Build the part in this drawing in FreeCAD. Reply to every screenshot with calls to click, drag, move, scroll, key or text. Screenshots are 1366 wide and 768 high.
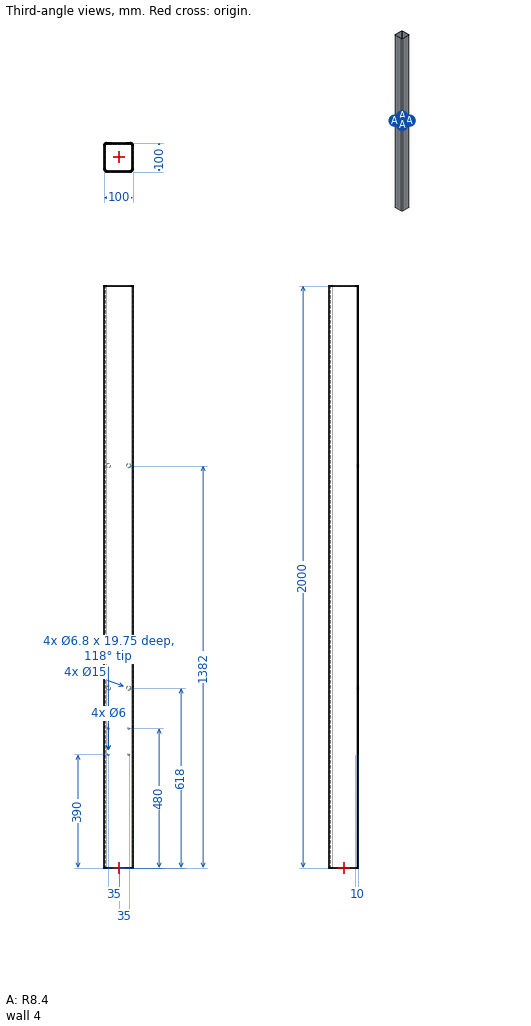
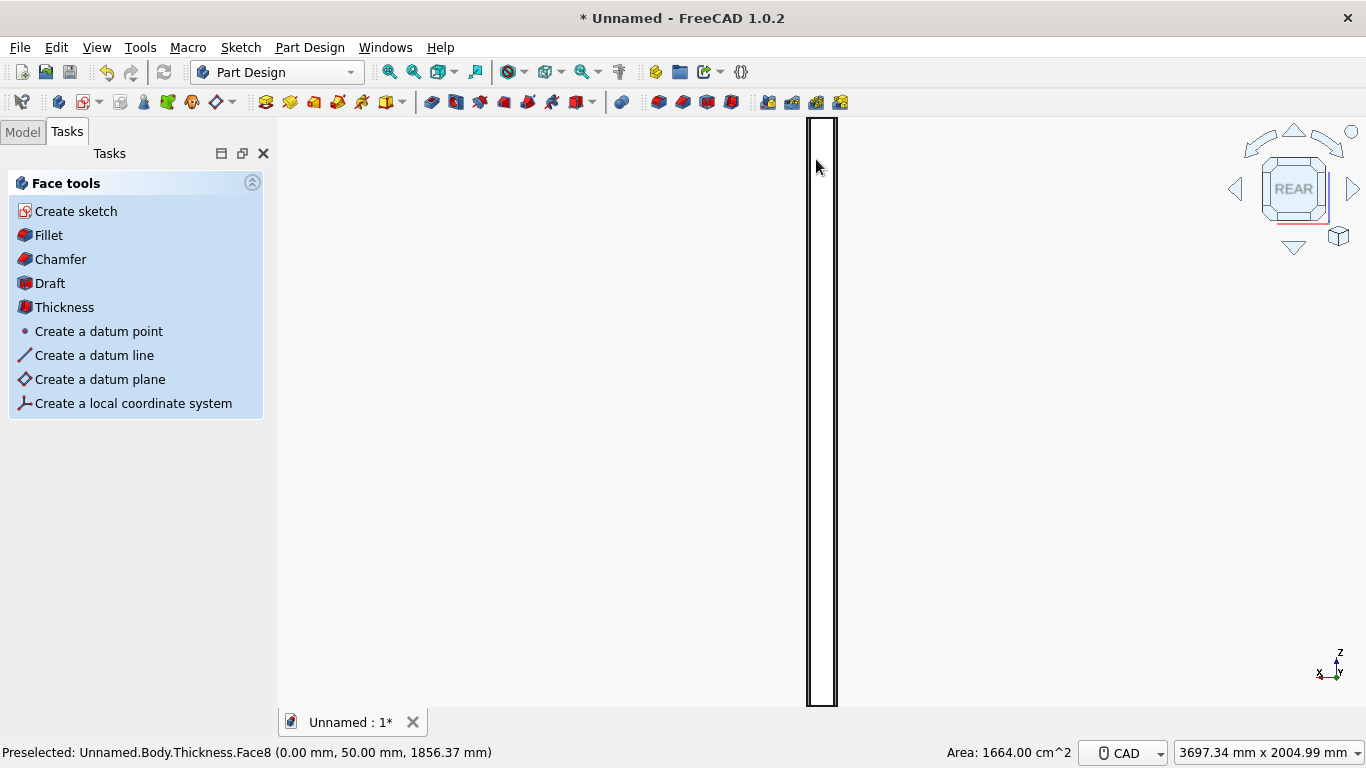
click(84, 102)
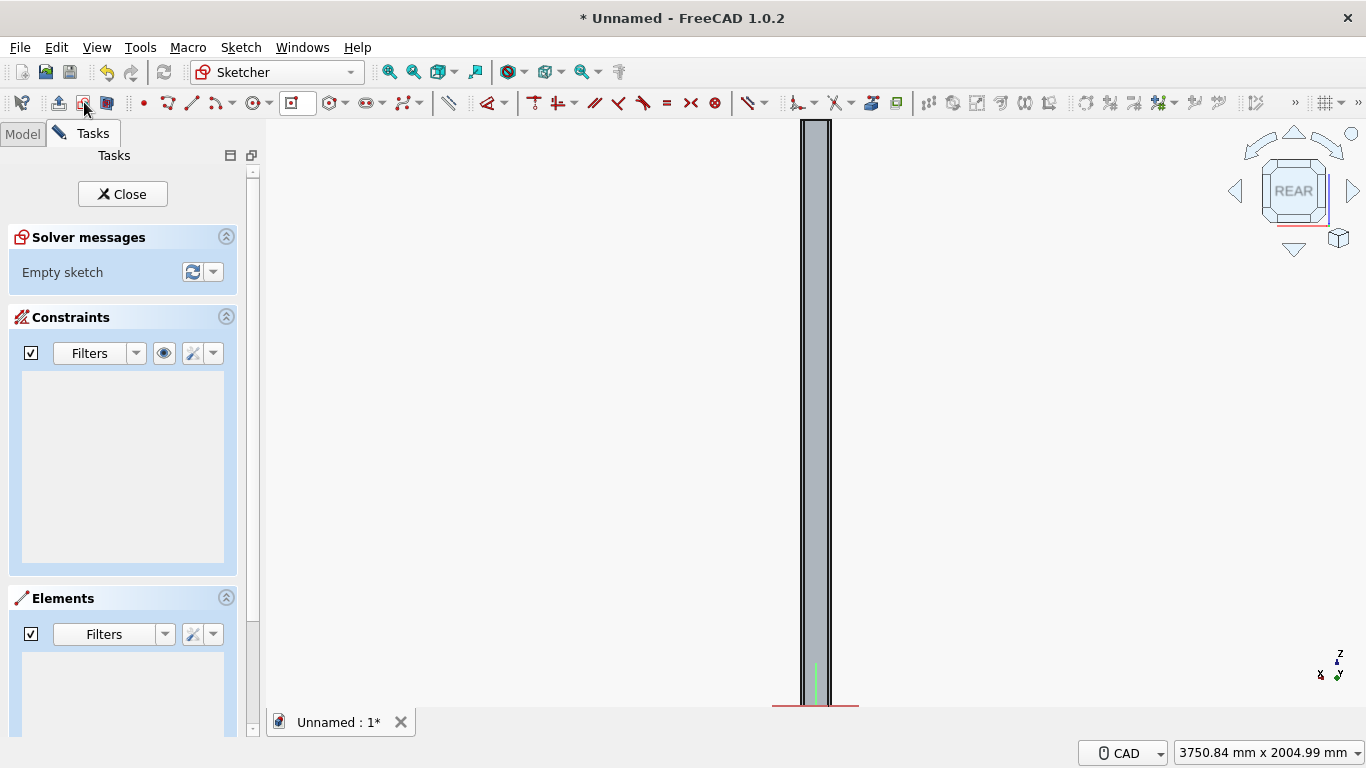
scroll(821, 592, up, 13)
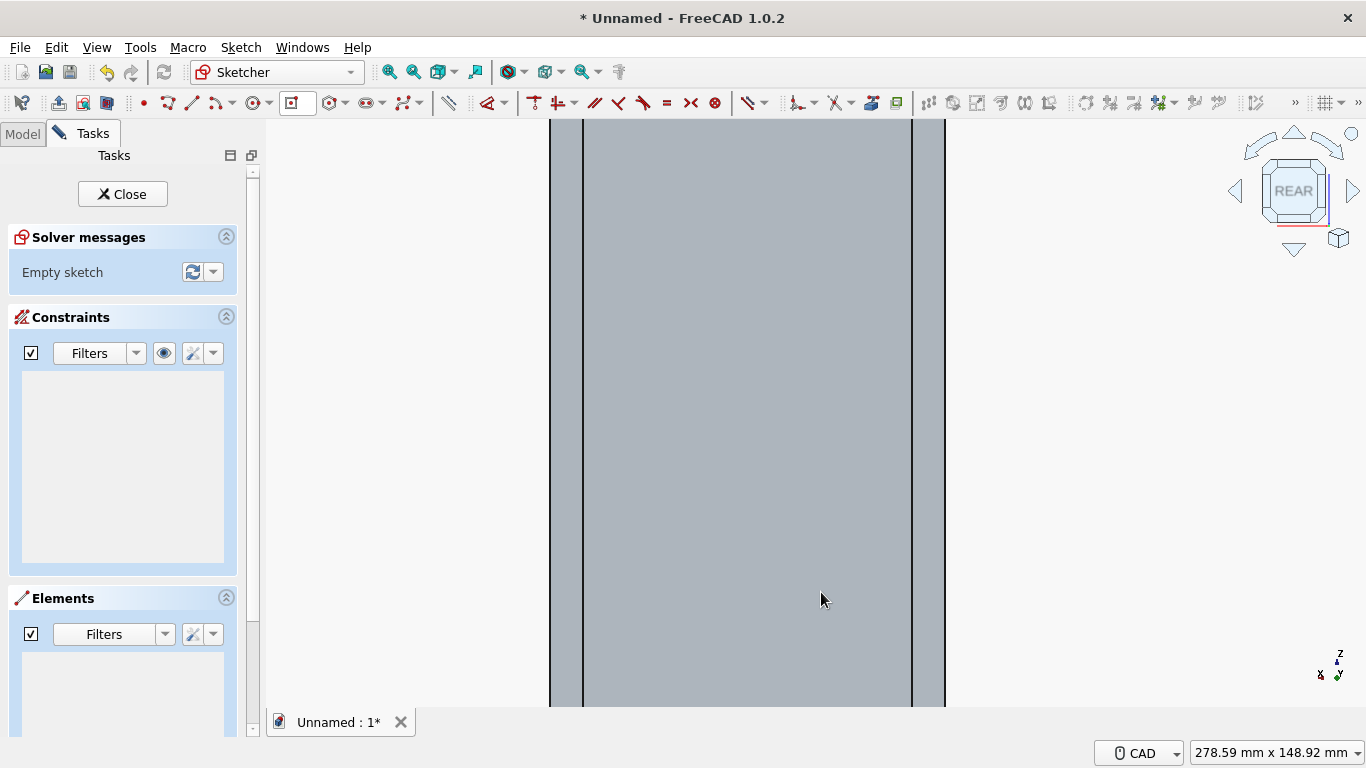
click(254, 104)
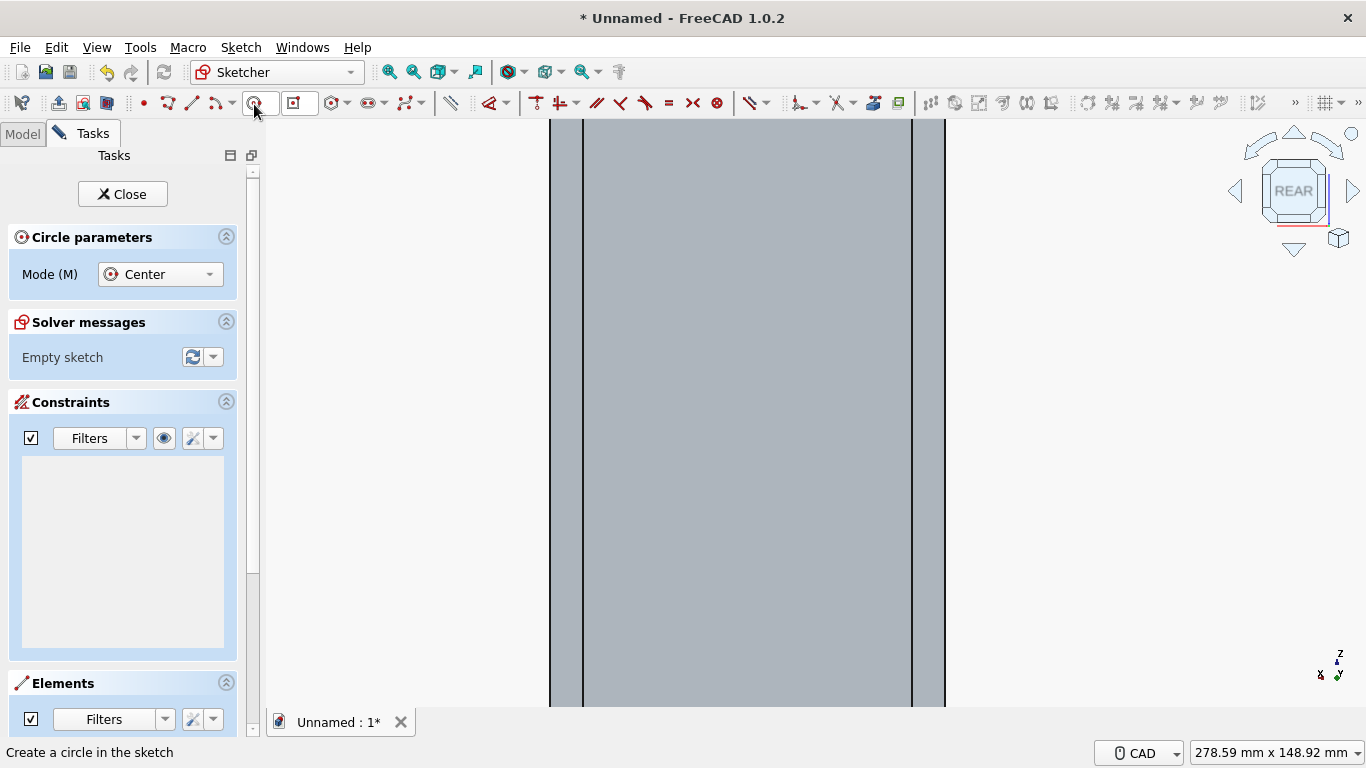
scroll(886, 581, up, 3)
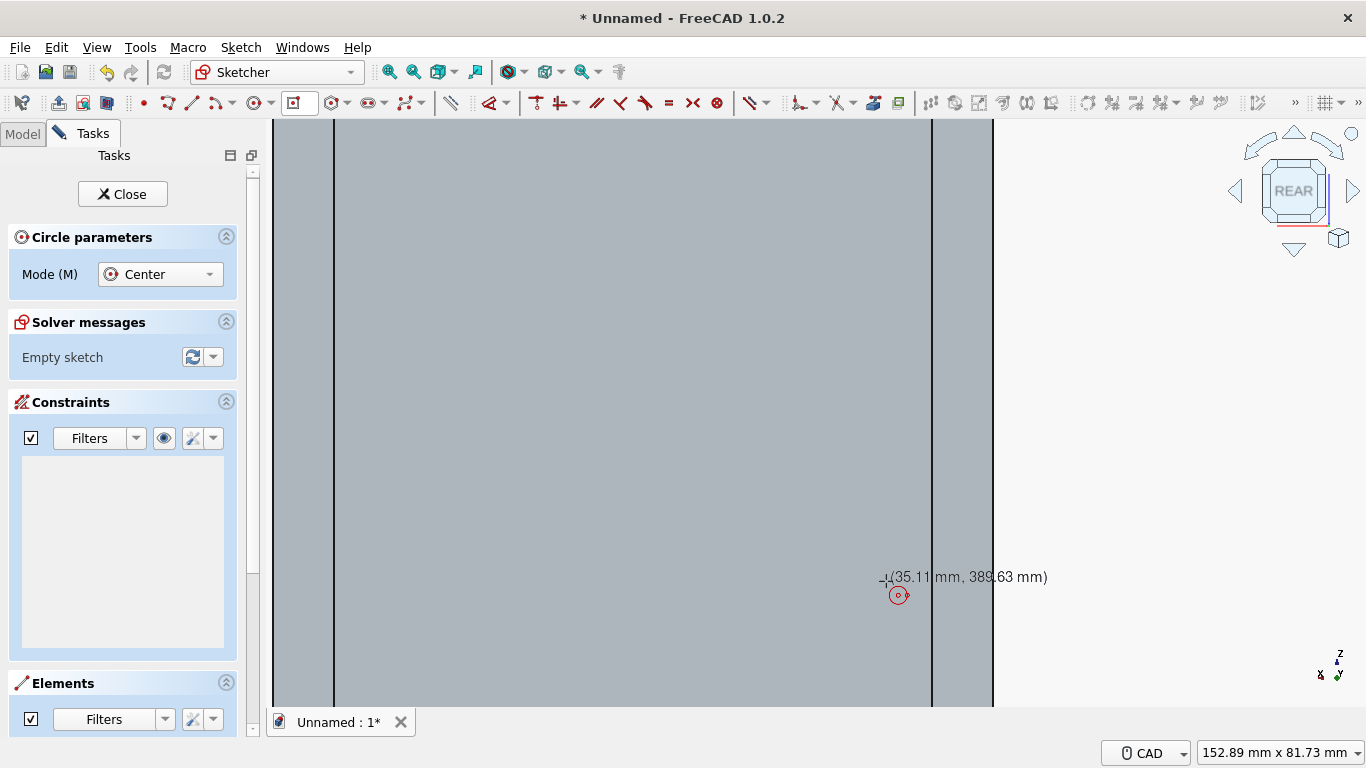
click(885, 579)
click(902, 562)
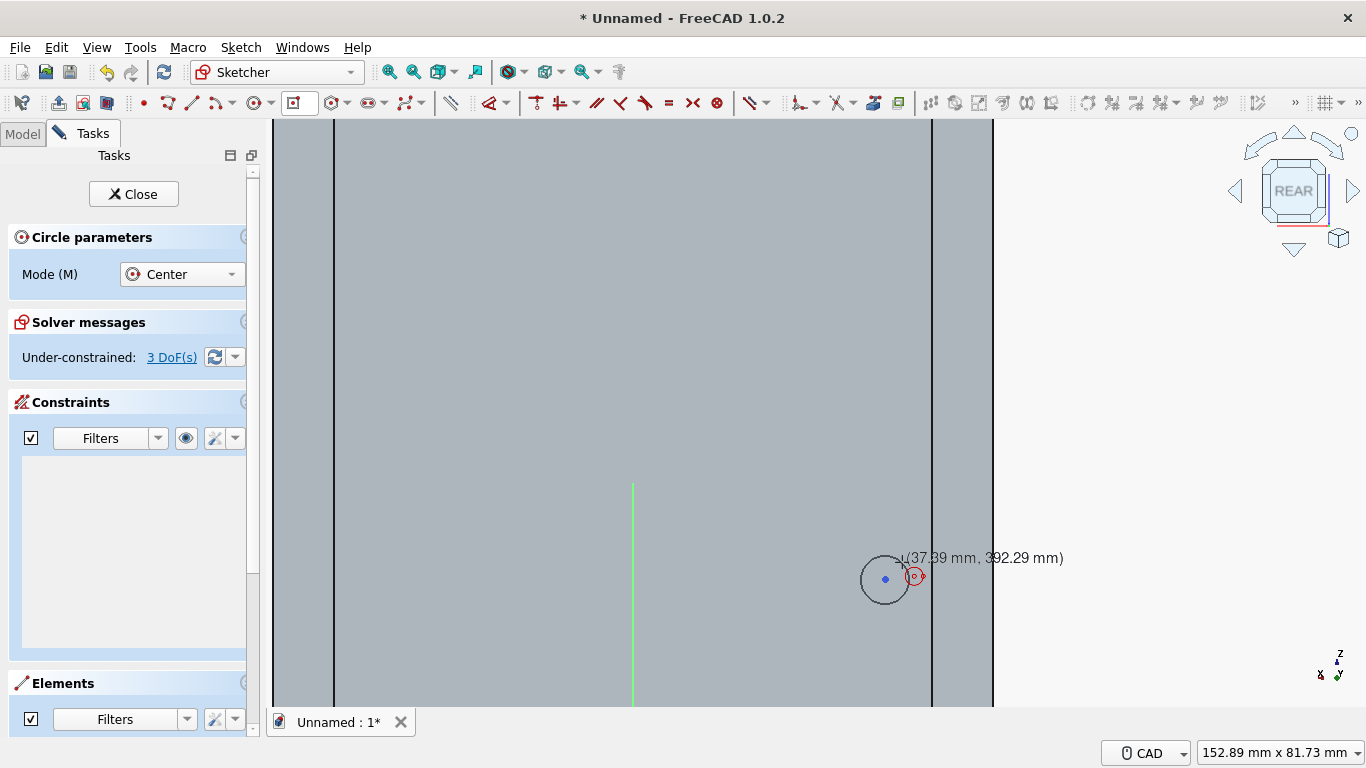
click(381, 579)
click(398, 562)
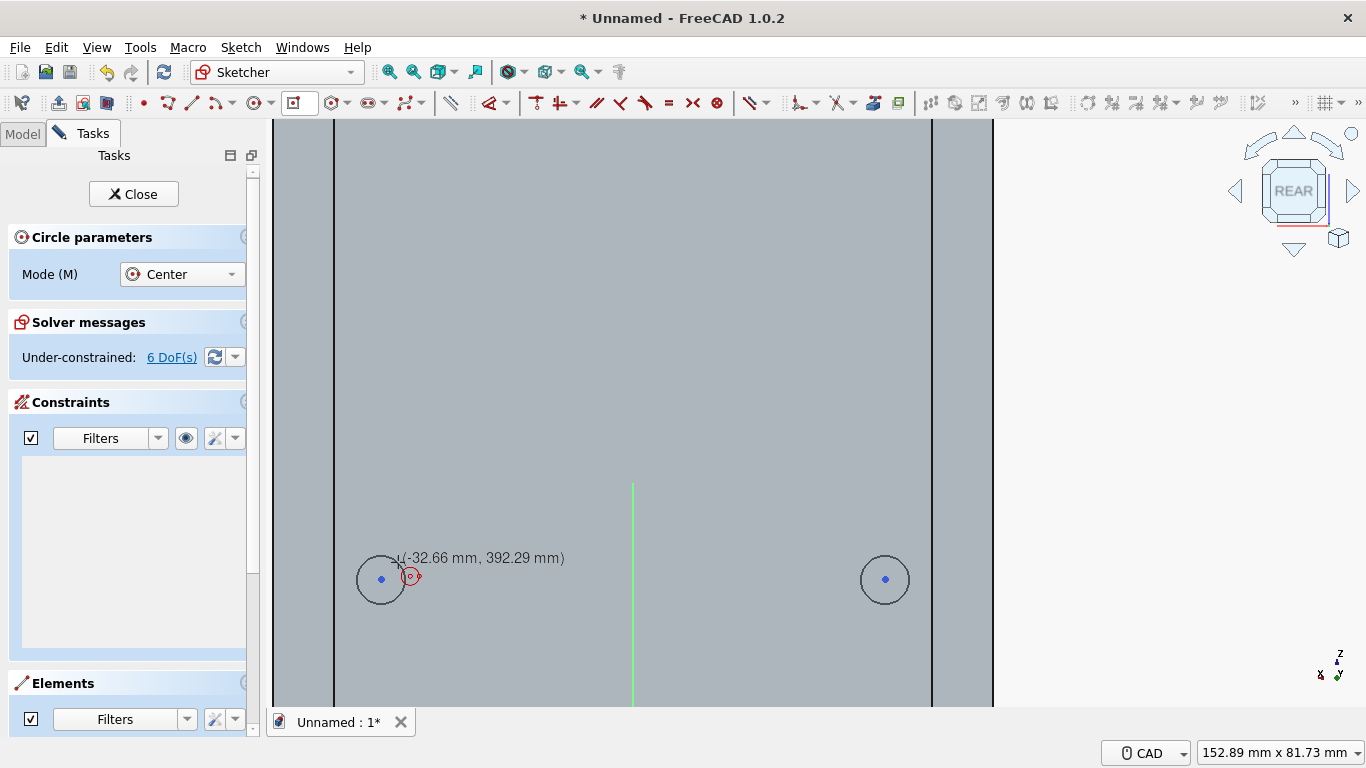
scroll(887, 604, down, 3)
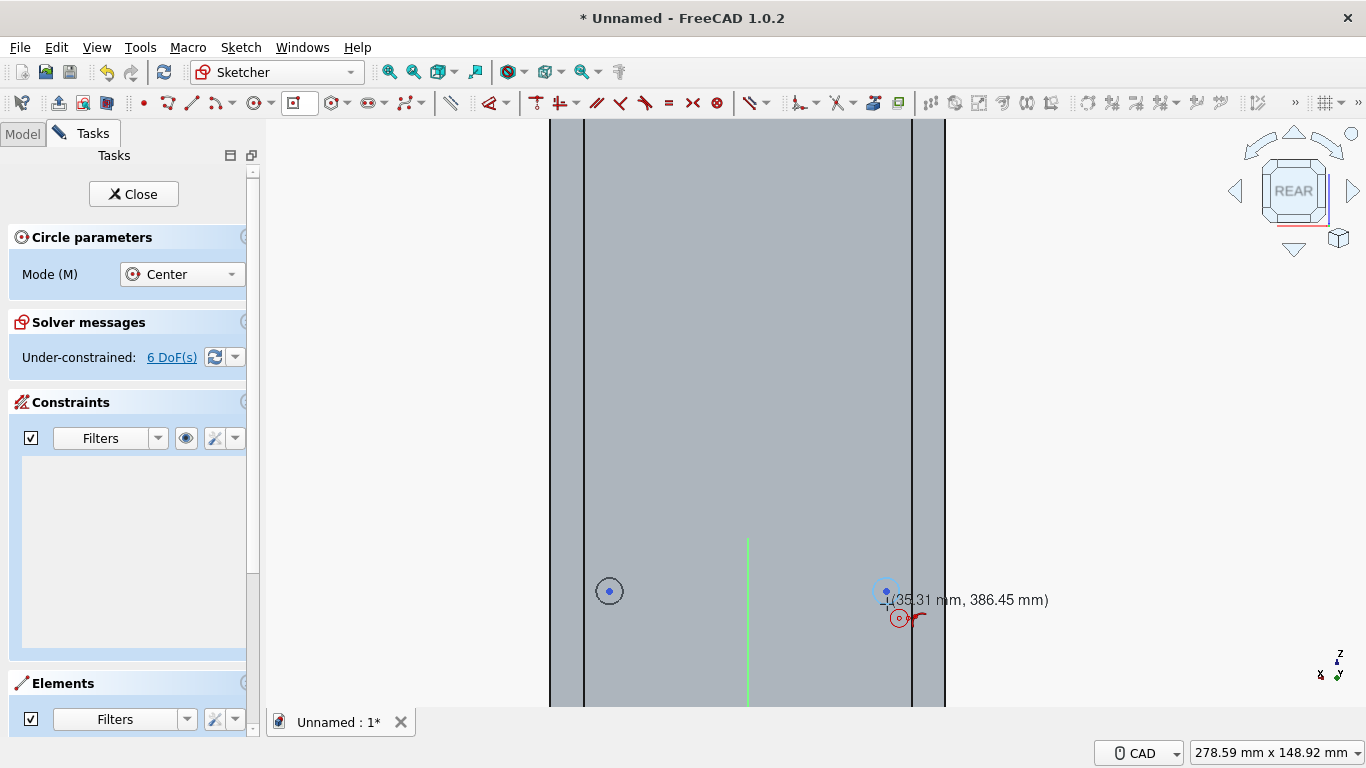
scroll(610, 236, up, 3)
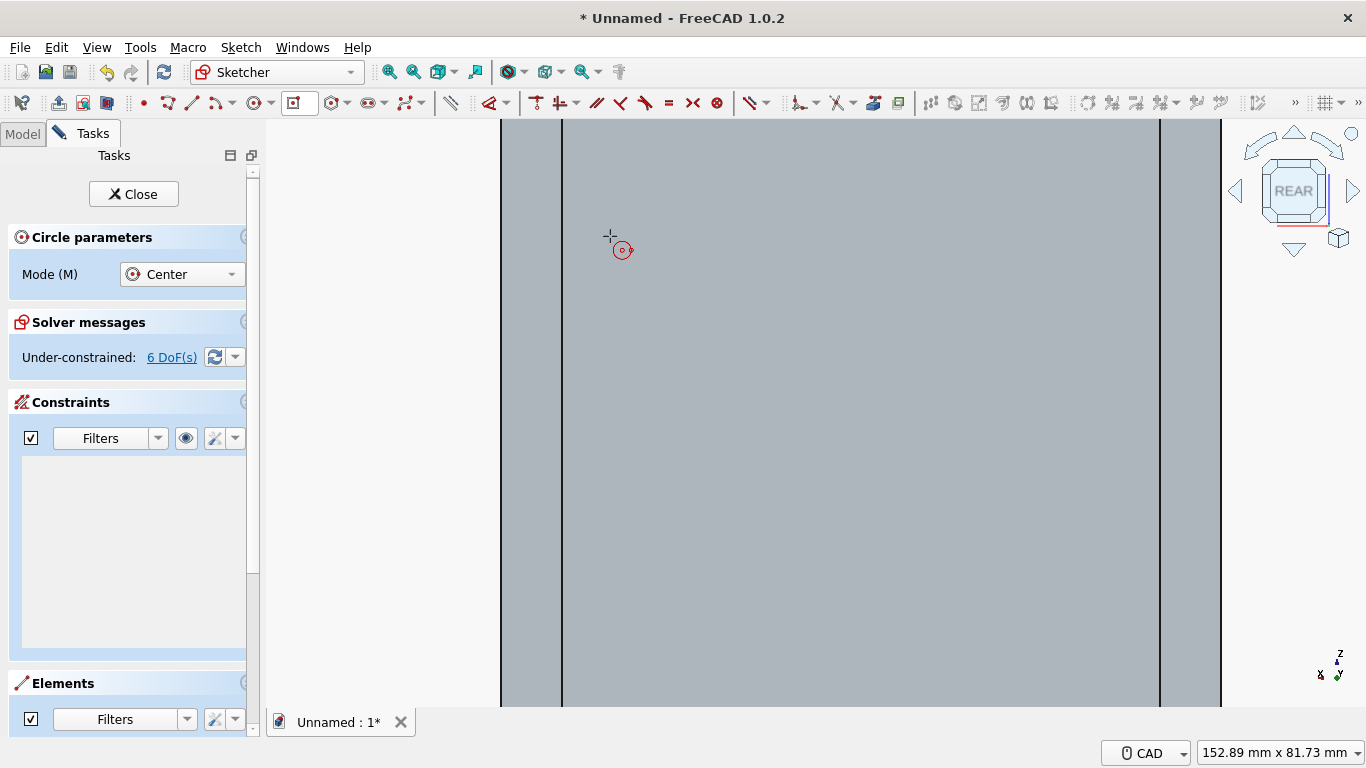
click(609, 235)
click(626, 218)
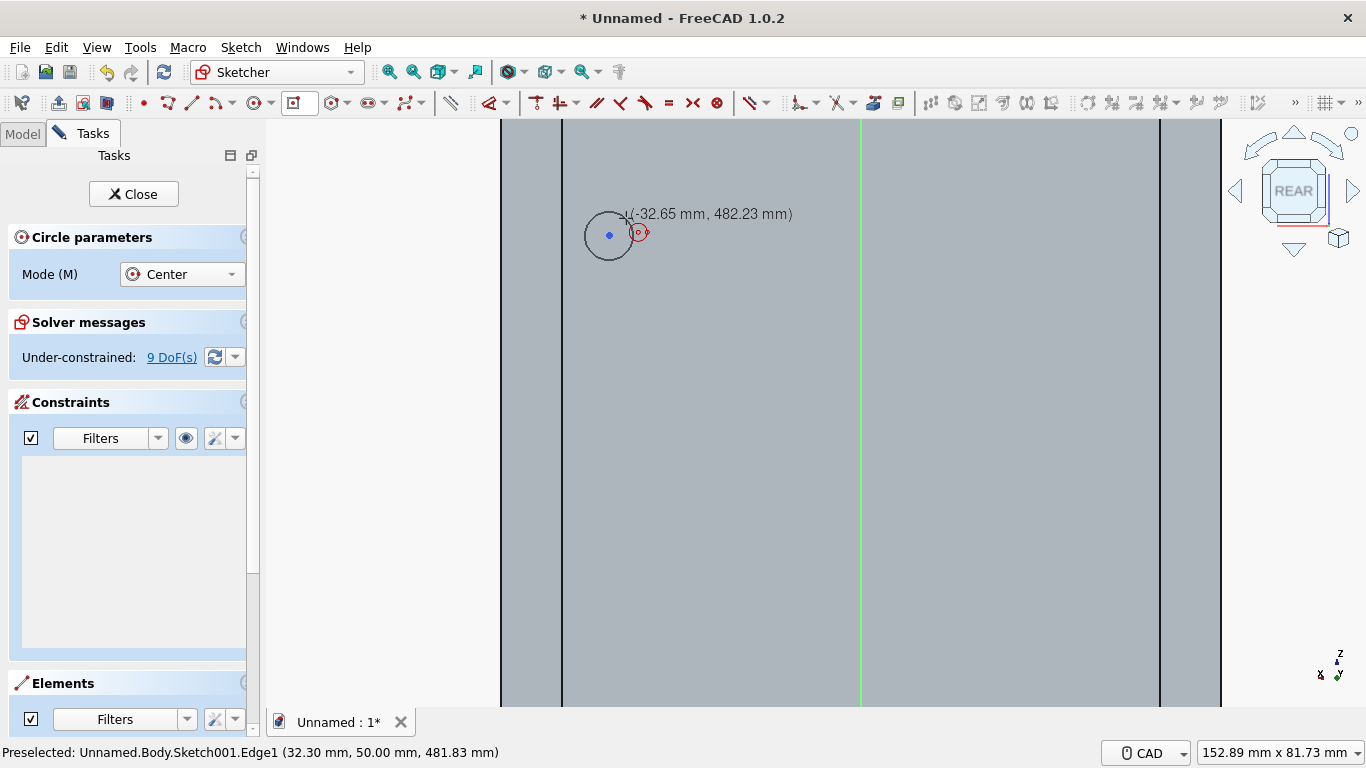
click(1113, 235)
click(1130, 218)
key(Escape)